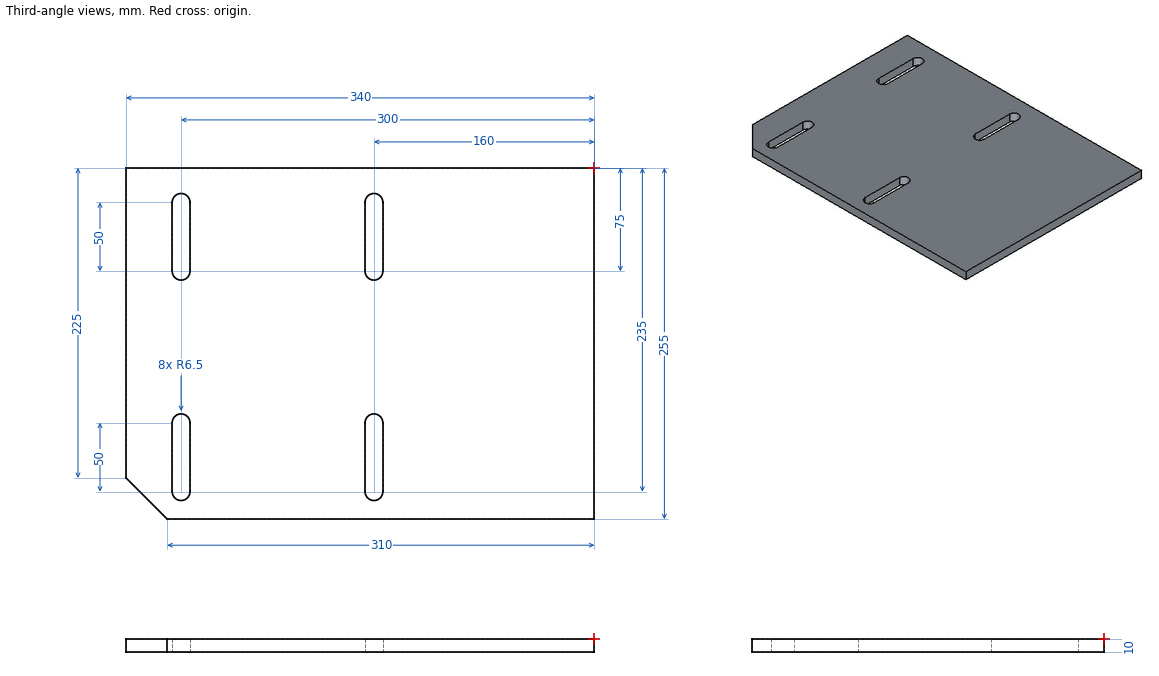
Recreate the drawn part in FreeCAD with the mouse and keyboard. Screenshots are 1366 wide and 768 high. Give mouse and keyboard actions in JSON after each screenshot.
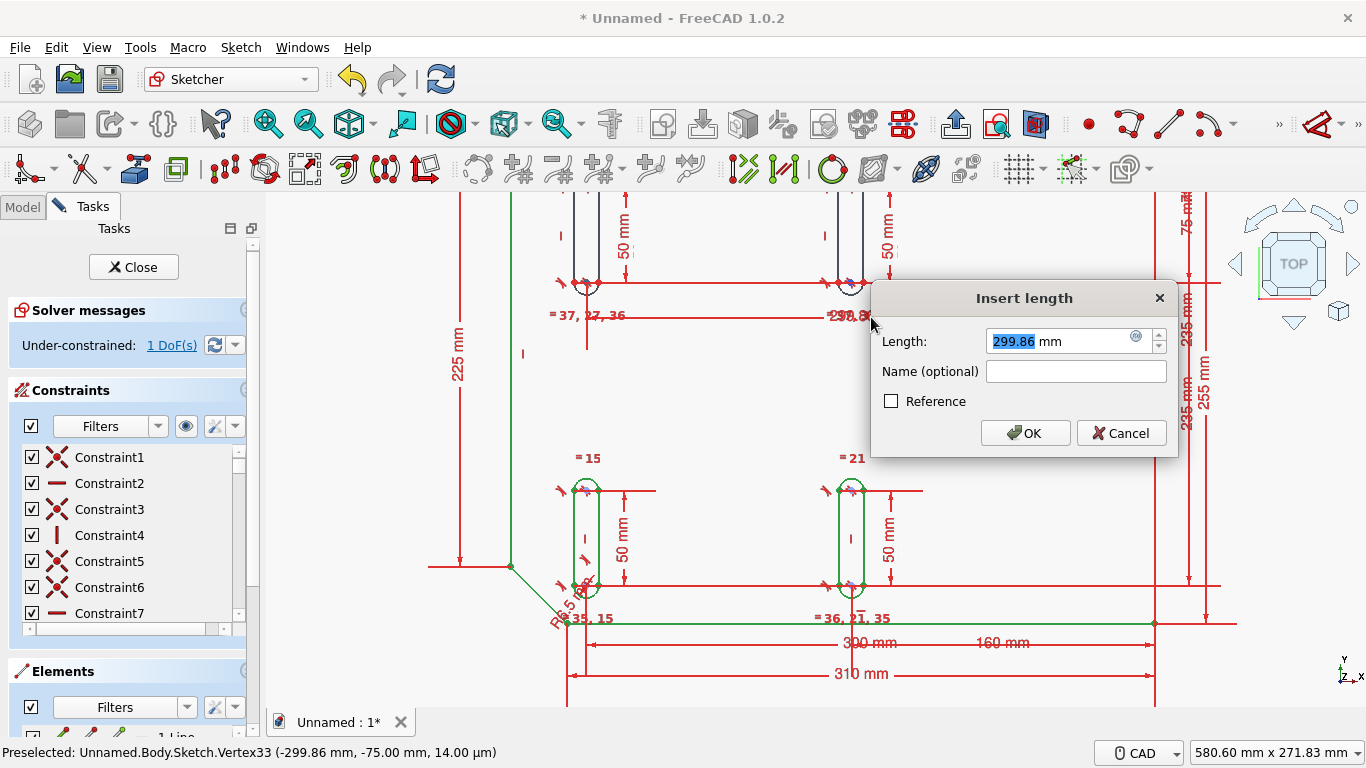
{"action": "type", "text": "300"}
{"action": "key", "text": "Return"}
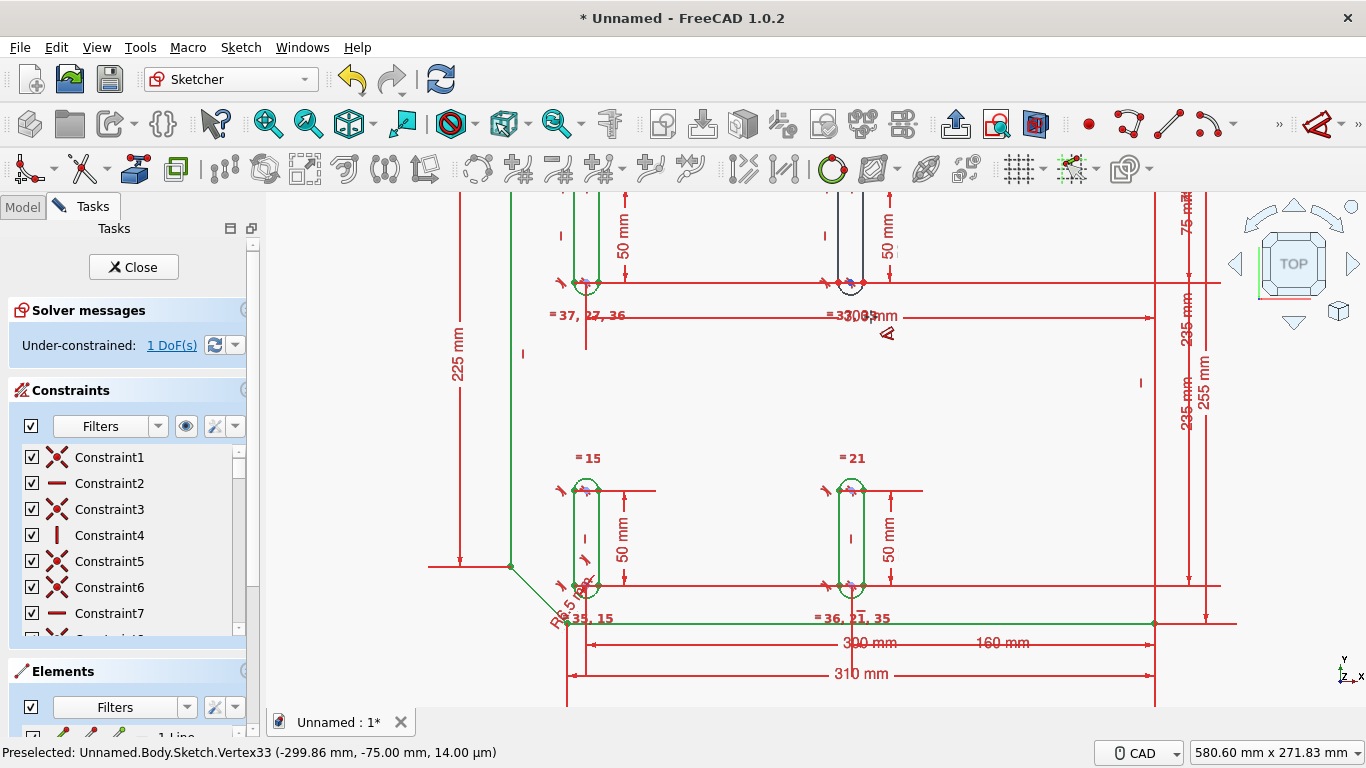
{"action": "left_click", "coordinate": [851, 283]}
{"action": "left_click", "coordinate": [1003, 317]}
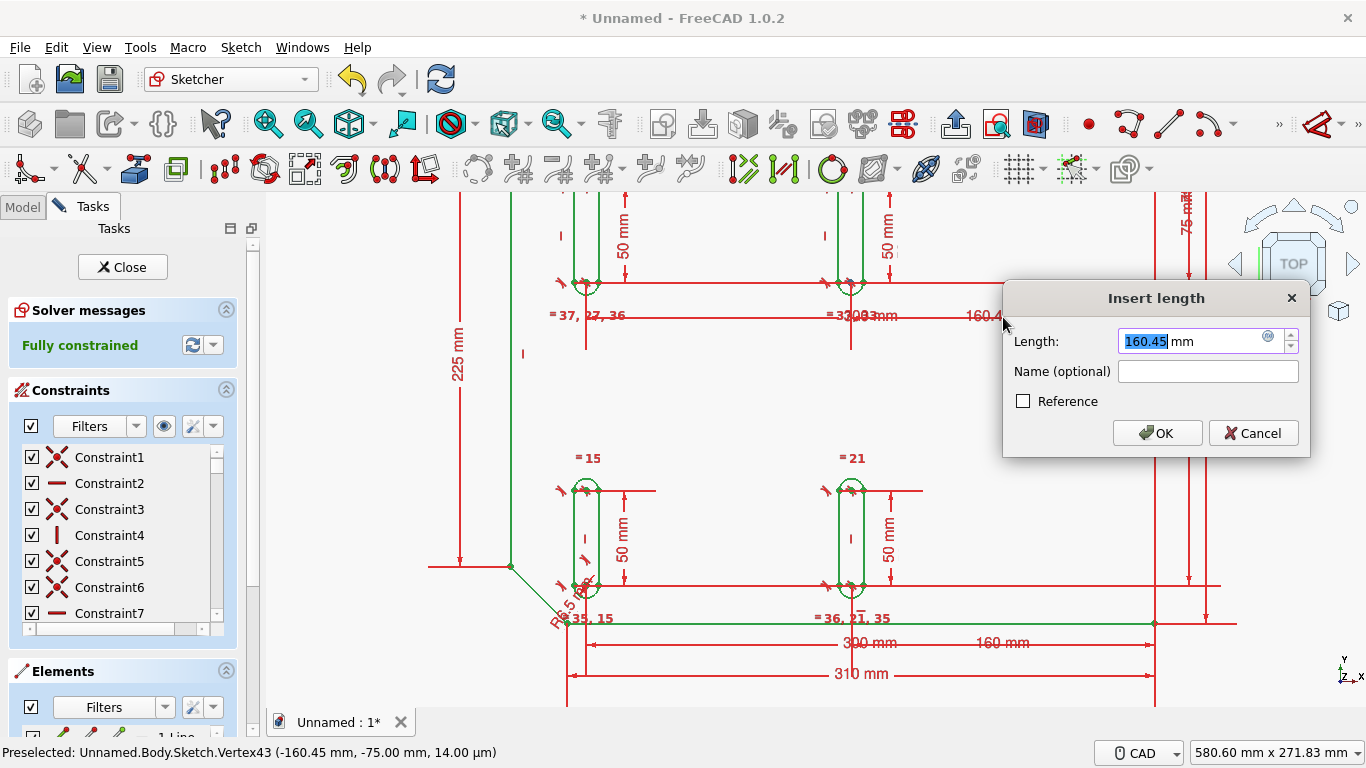
{"action": "type", "text": "160"}
{"action": "key", "text": "Return"}
{"action": "key", "text": "Escape"}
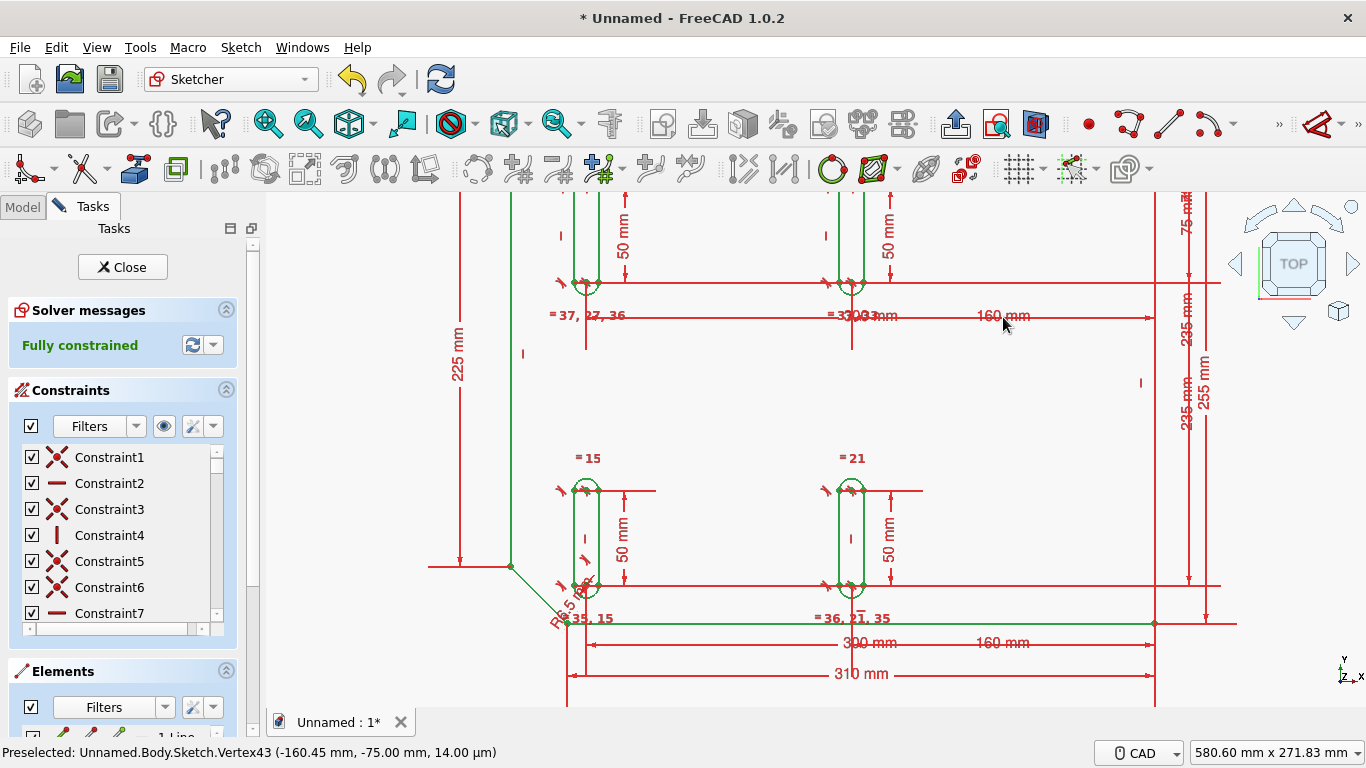
{"action": "left_click", "coordinate": [123, 267]}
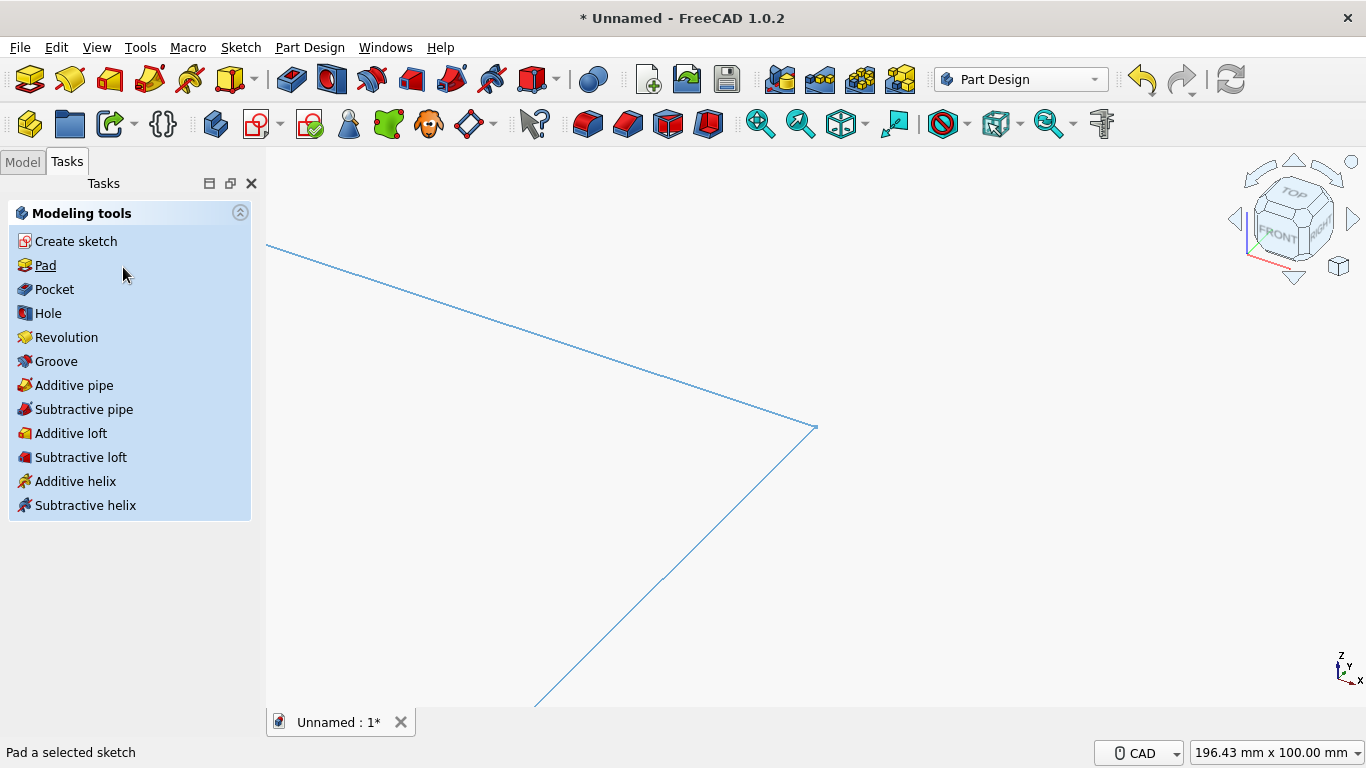
{"action": "left_click", "coordinate": [30, 80]}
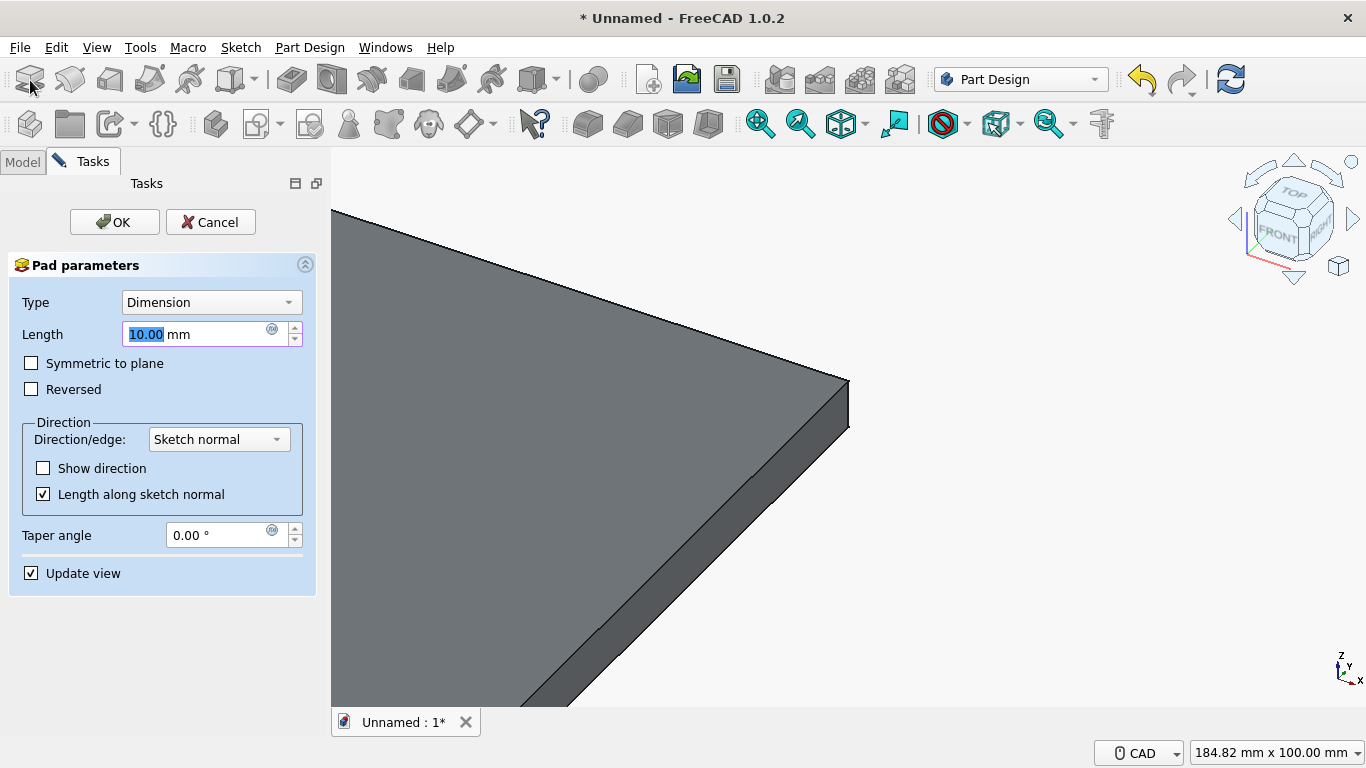
{"action": "type", "text": "10"}
{"action": "key", "text": "Tab"}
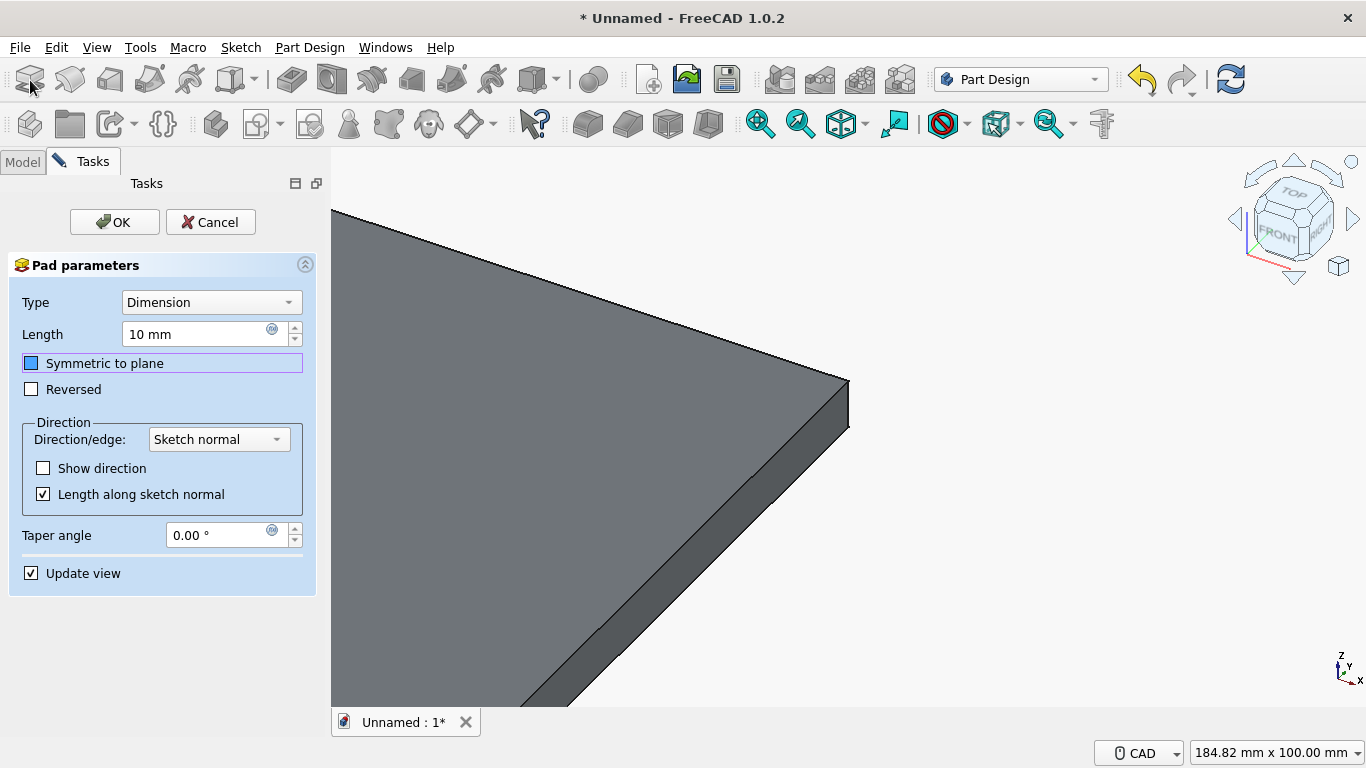
{"action": "left_click", "coordinate": [30, 389]}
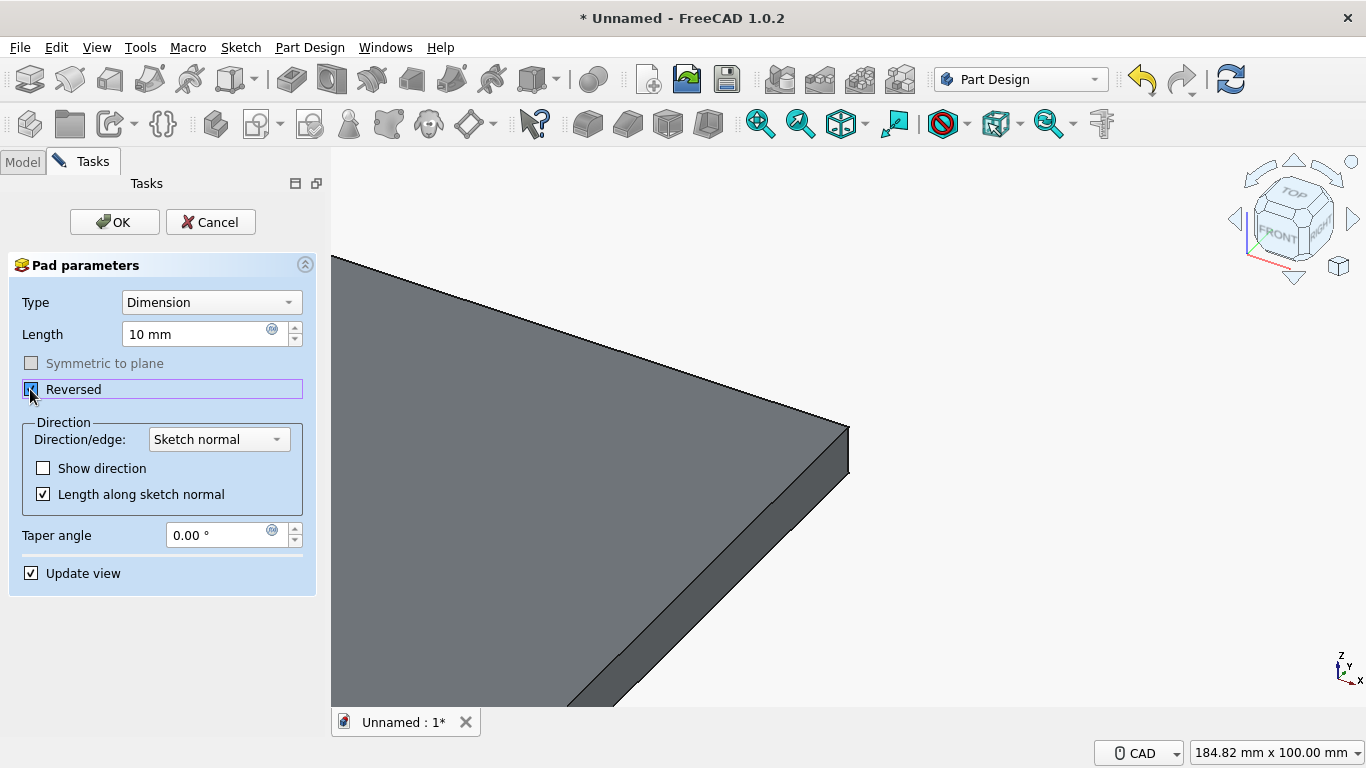
{"action": "left_click", "coordinate": [115, 222]}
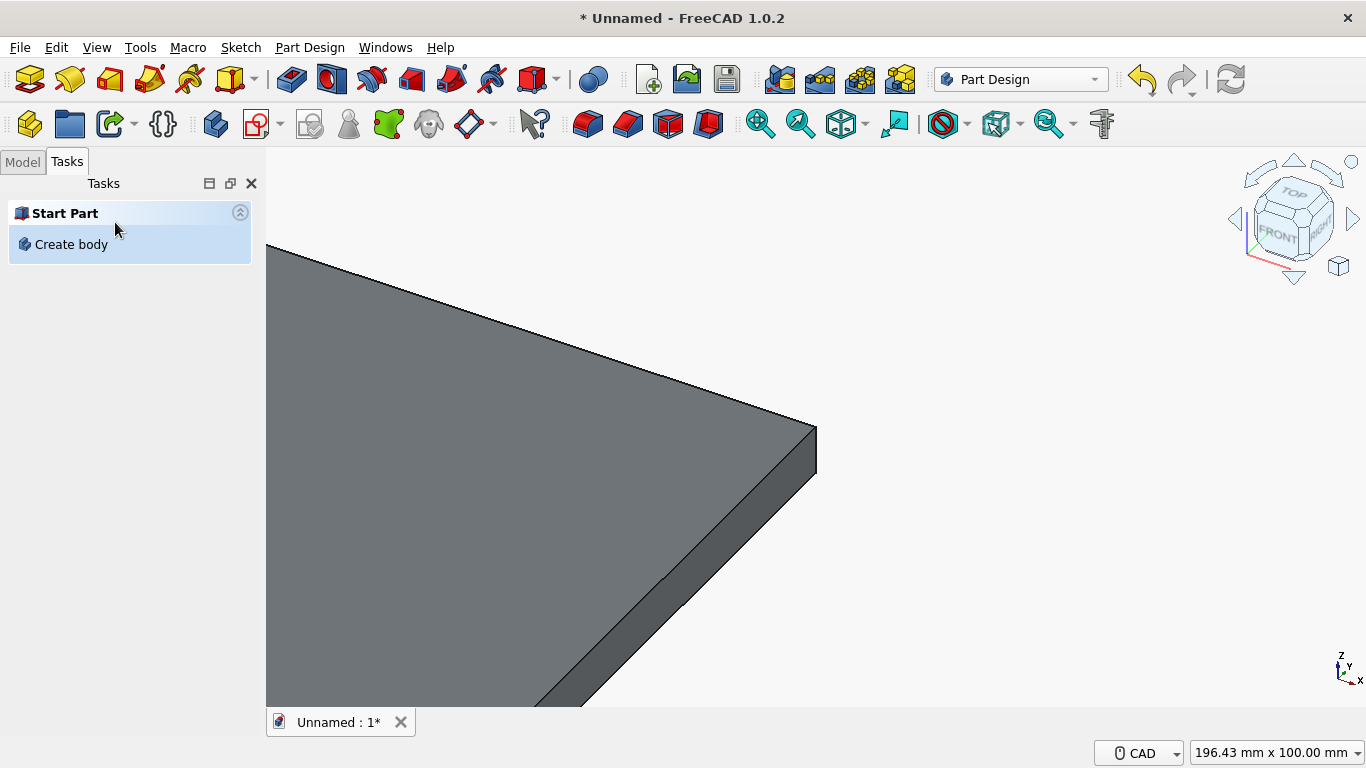
{"action": "key", "text": "0"}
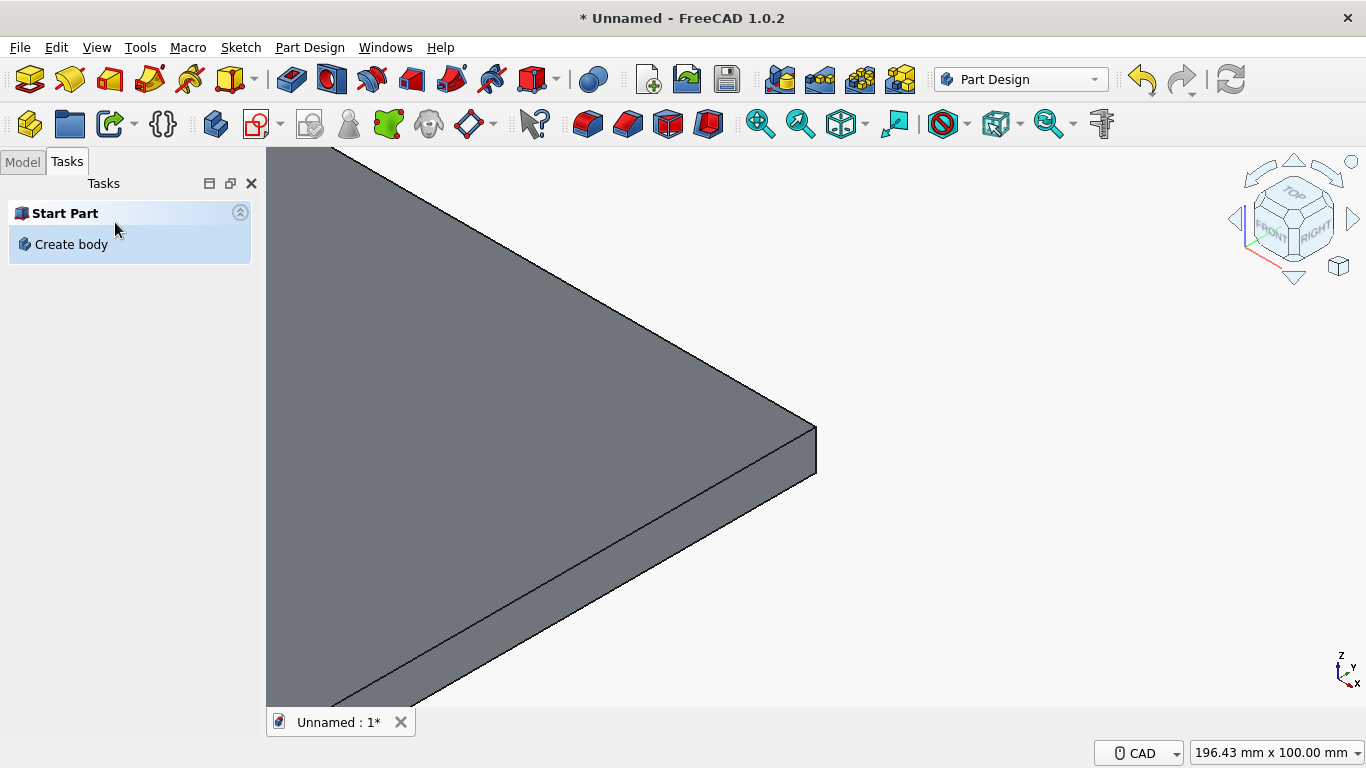
{"action": "key", "text": "v f"}